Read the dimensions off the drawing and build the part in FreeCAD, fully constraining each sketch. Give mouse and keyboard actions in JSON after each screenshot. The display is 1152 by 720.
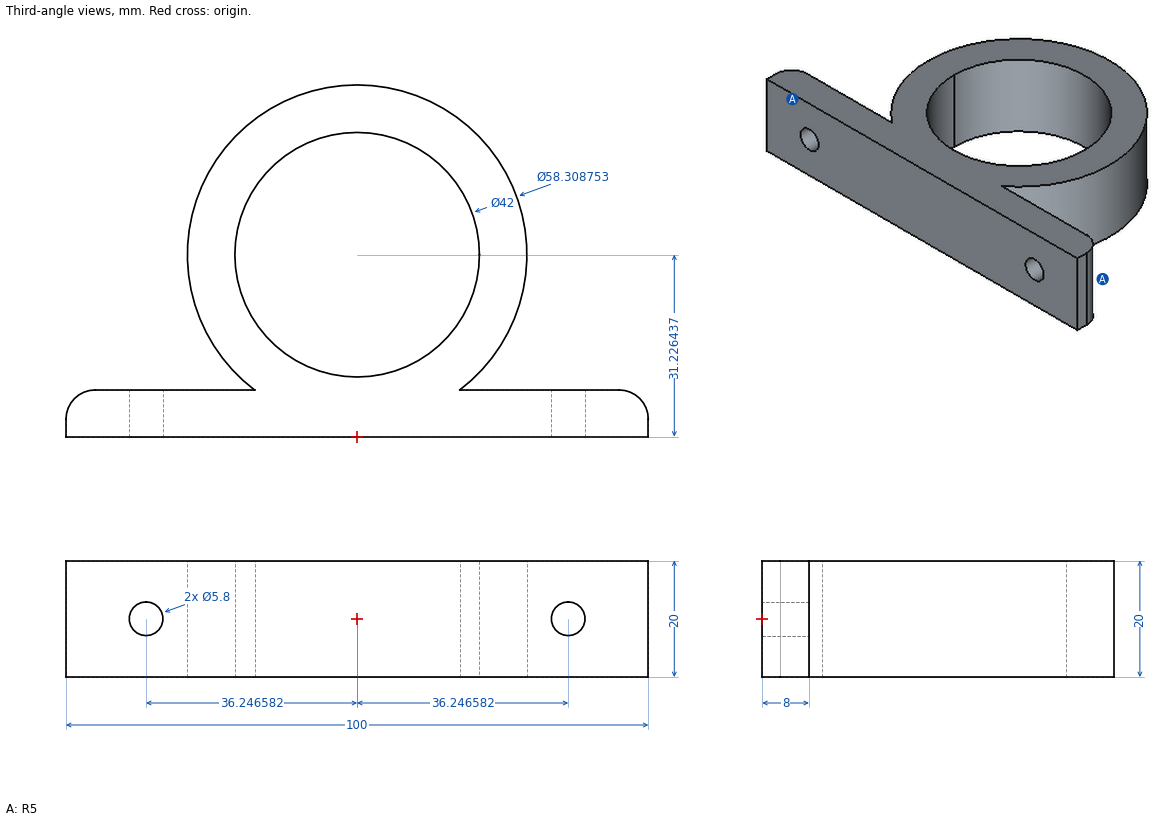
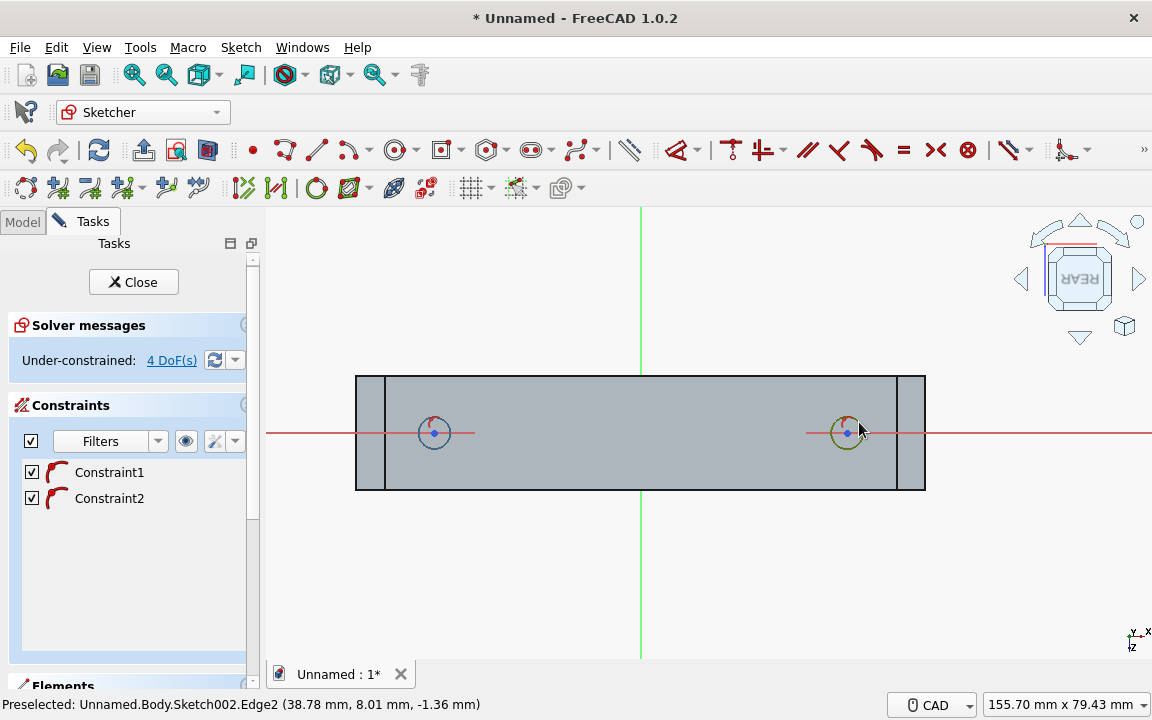
{"action": "left_click", "coordinate": [904, 150]}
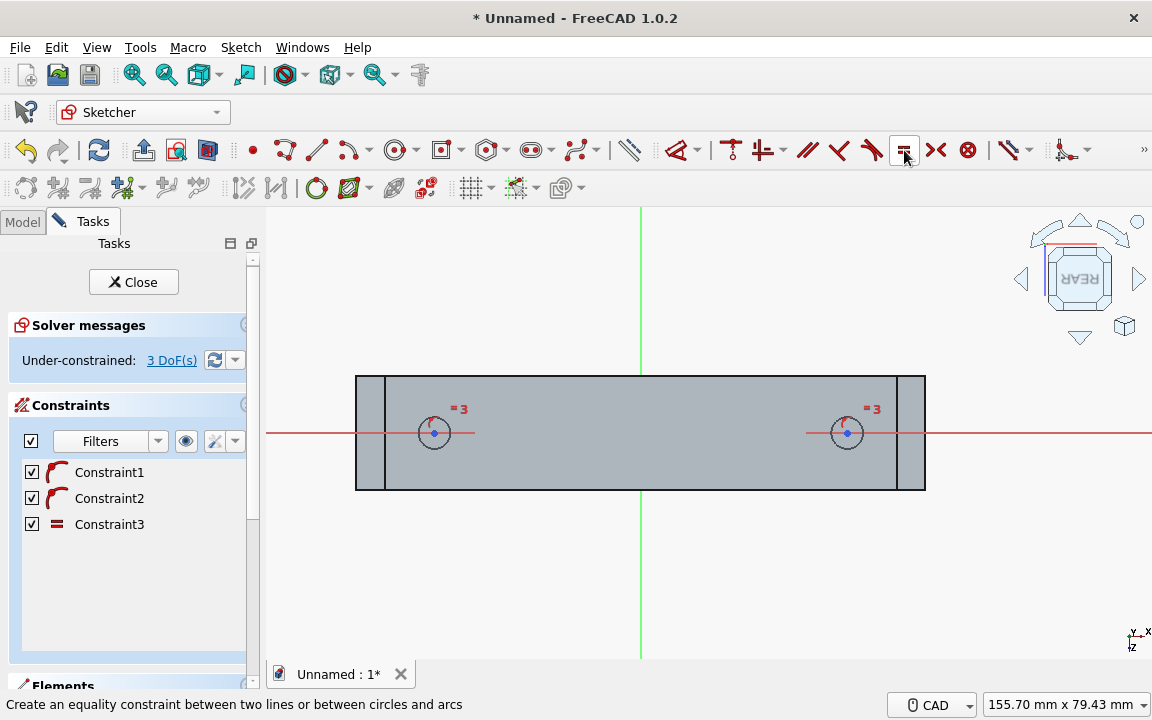
{"action": "left_click", "coordinate": [676, 150]}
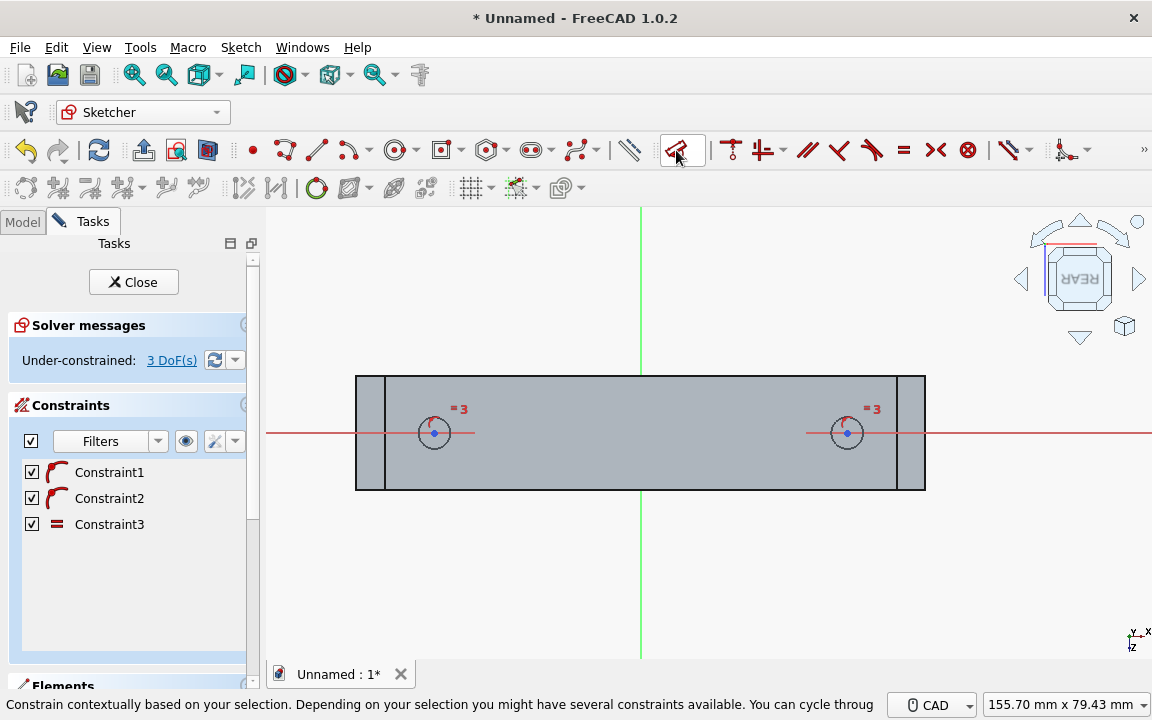
{"action": "scroll", "coordinate": [446, 422], "scroll_direction": "up", "scroll_amount": 2}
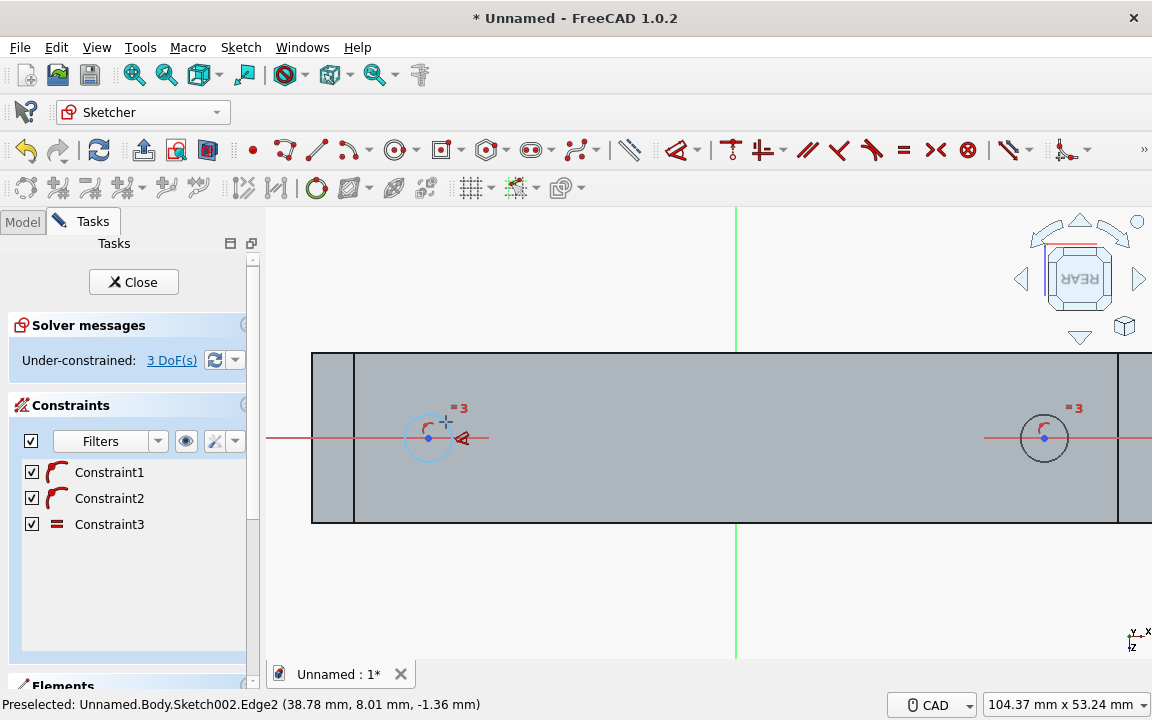
{"action": "left_click", "coordinate": [445, 422]}
{"action": "left_click", "coordinate": [468, 399]}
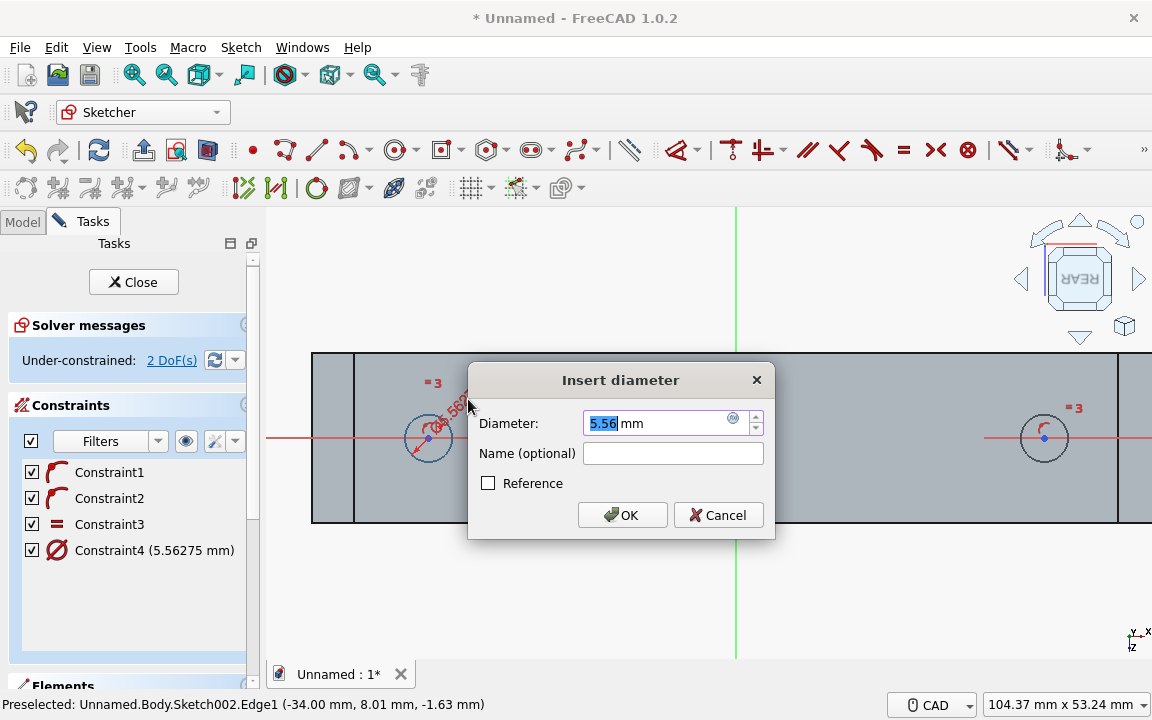
{"action": "type", "text": "5.8"}
{"action": "key", "text": "Return"}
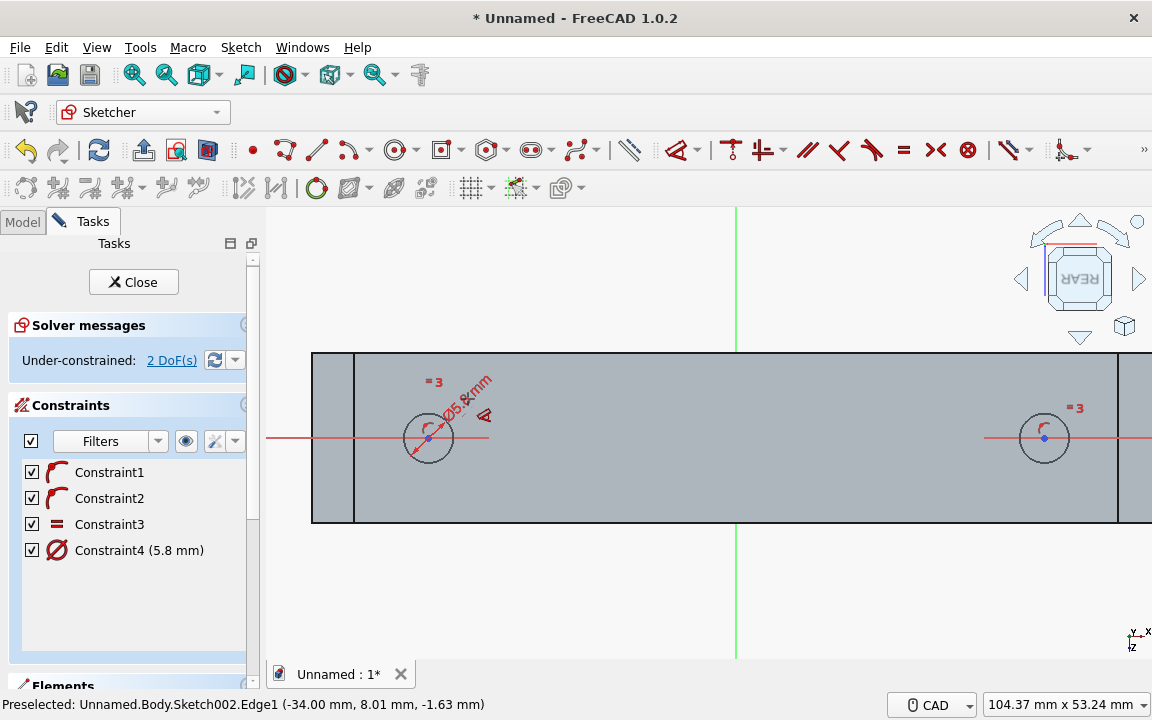
{"action": "left_click", "coordinate": [429, 438]}
{"action": "left_click", "coordinate": [582, 472]}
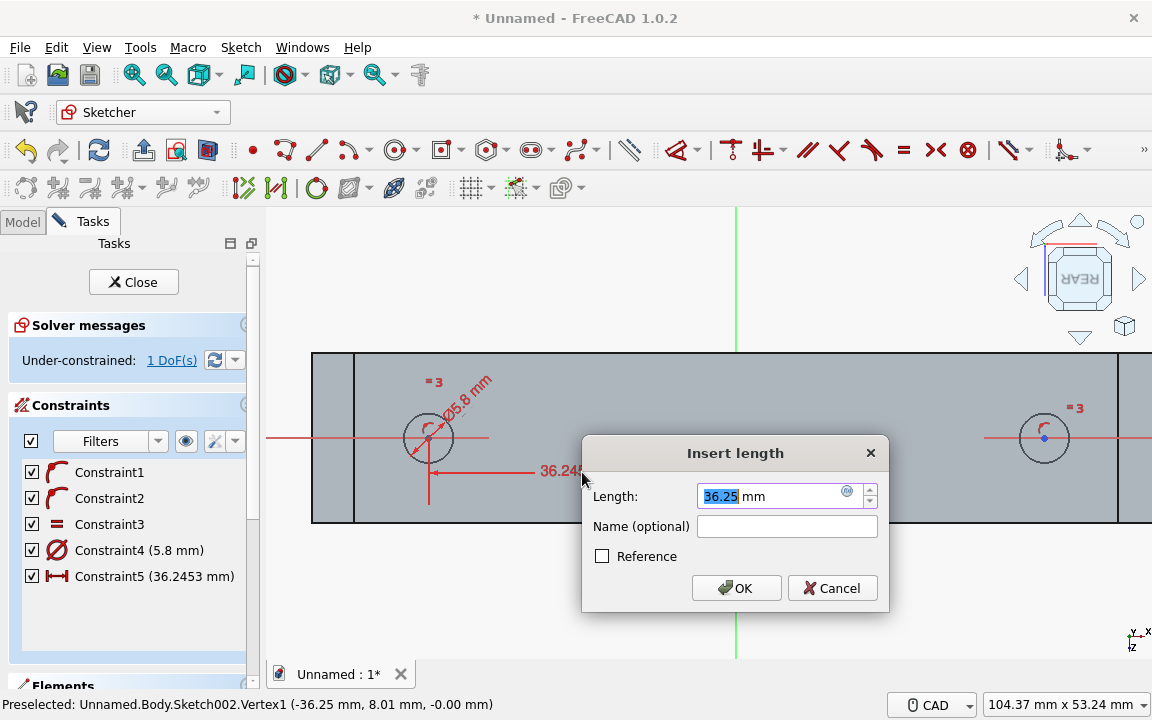
{"action": "type", "text": "36.246582"}
{"action": "key", "text": "Return"}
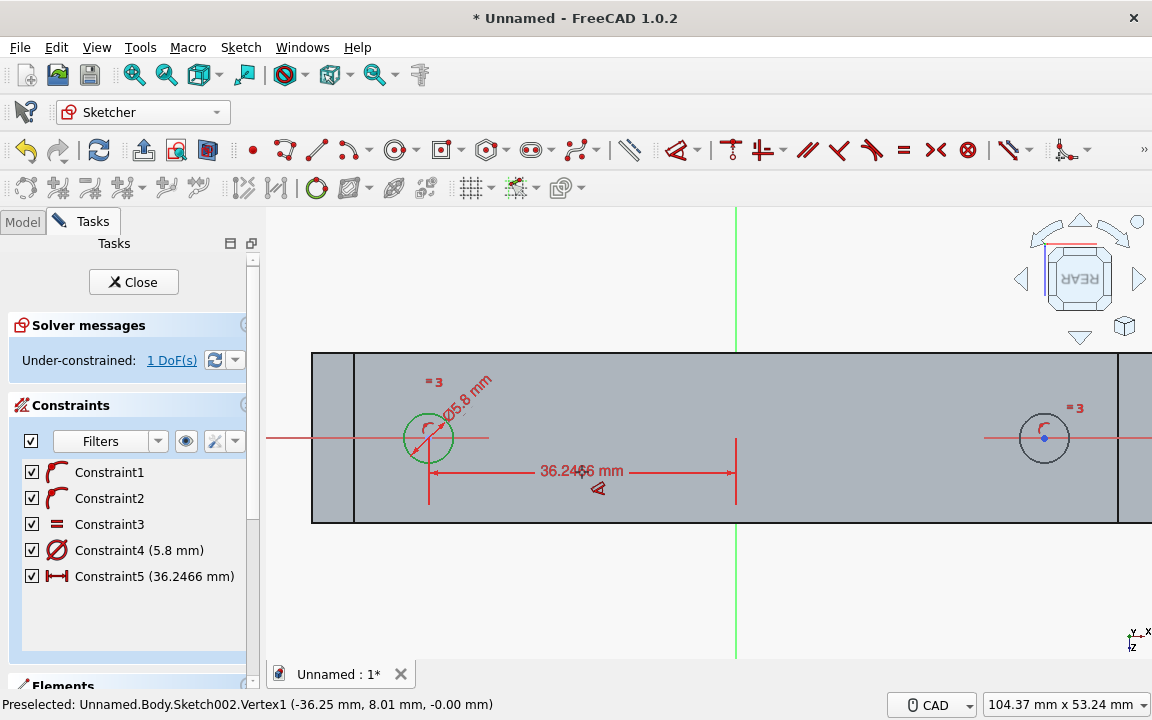
{"action": "scroll", "coordinate": [446, 422], "scroll_direction": "down", "scroll_amount": 2}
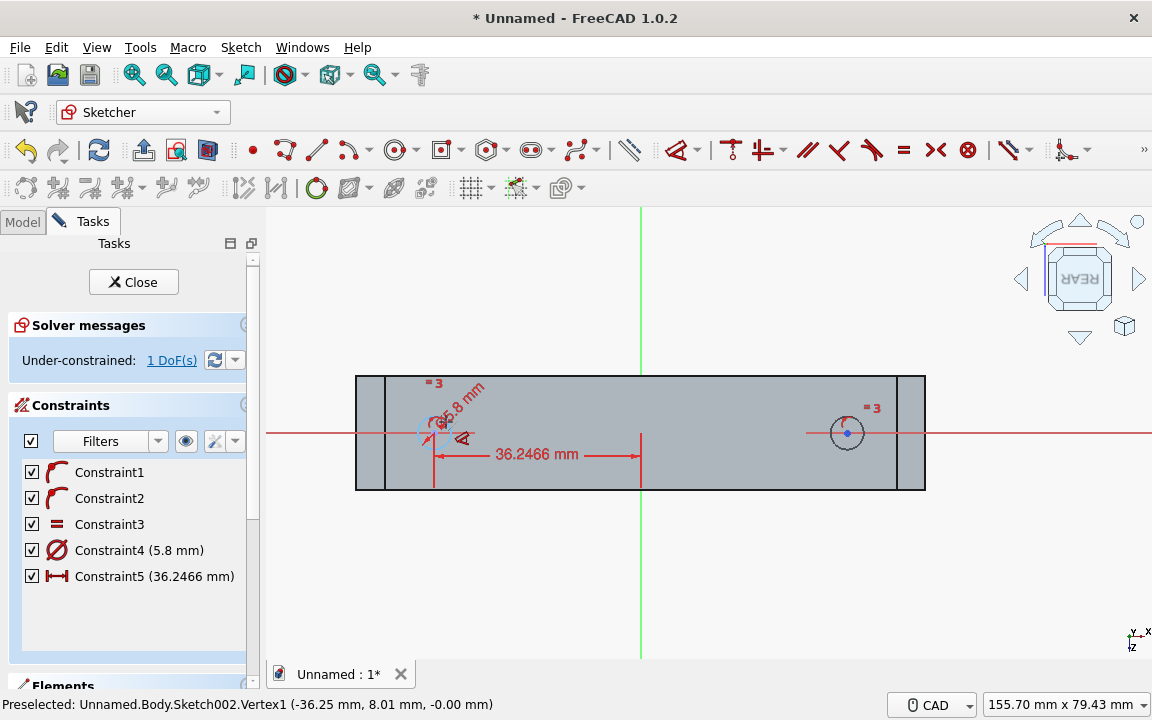
{"action": "left_click", "coordinate": [847, 433]}
{"action": "left_click", "coordinate": [744, 467]}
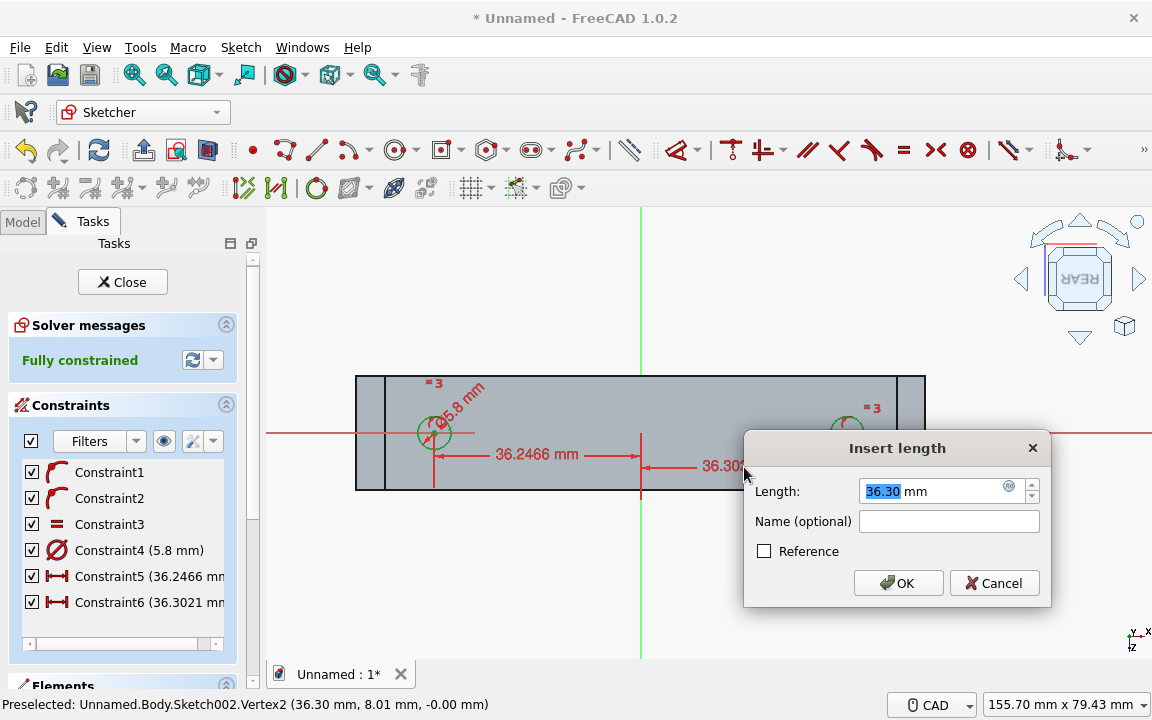
{"action": "type", "text": "36.246582"}
{"action": "key", "text": "Return"}
{"action": "key", "text": "Escape"}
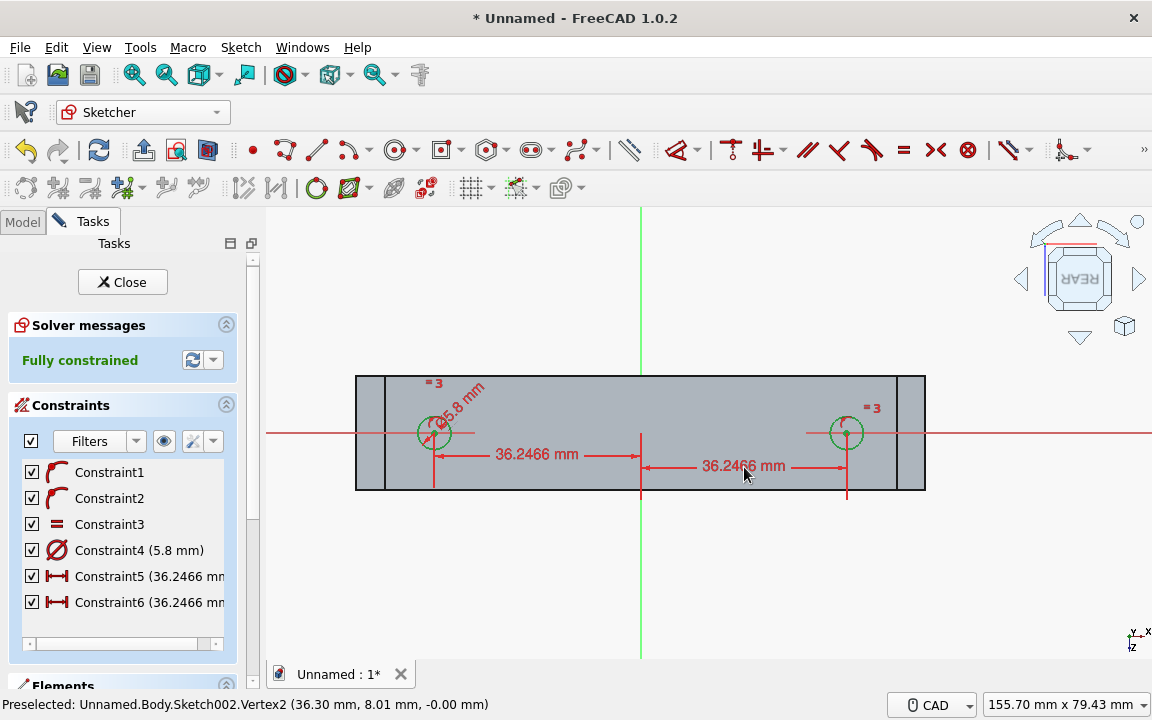
{"action": "left_click", "coordinate": [123, 282]}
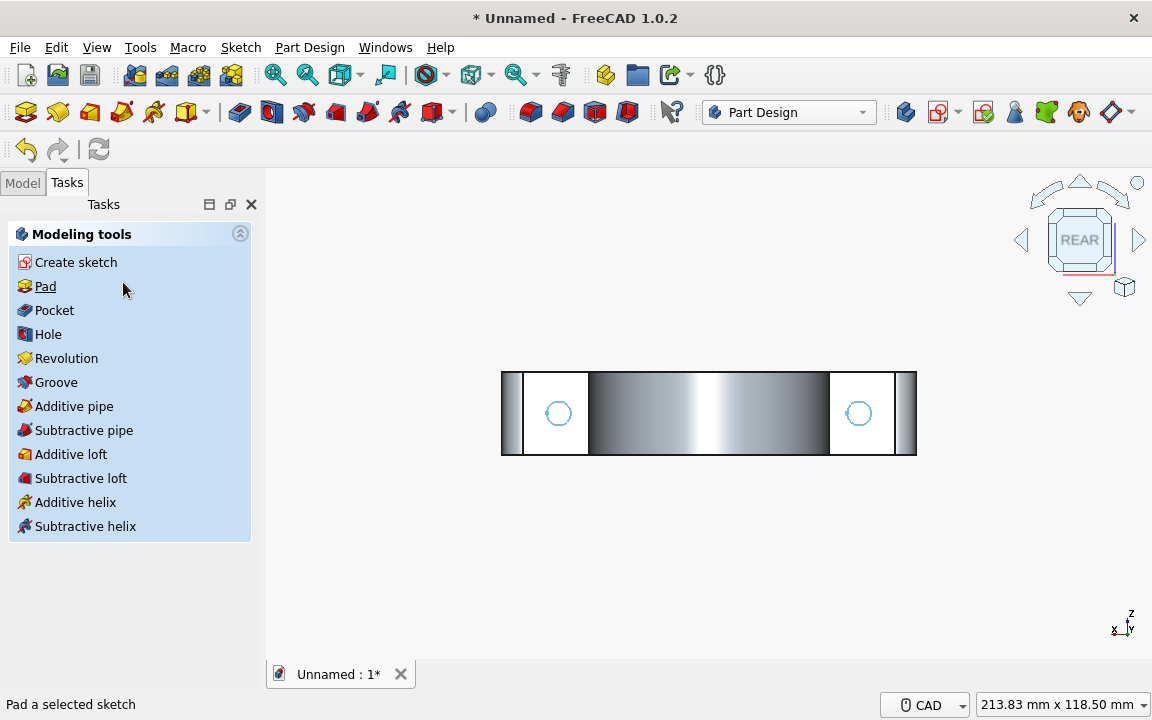
{"action": "left_click", "coordinate": [240, 112]}